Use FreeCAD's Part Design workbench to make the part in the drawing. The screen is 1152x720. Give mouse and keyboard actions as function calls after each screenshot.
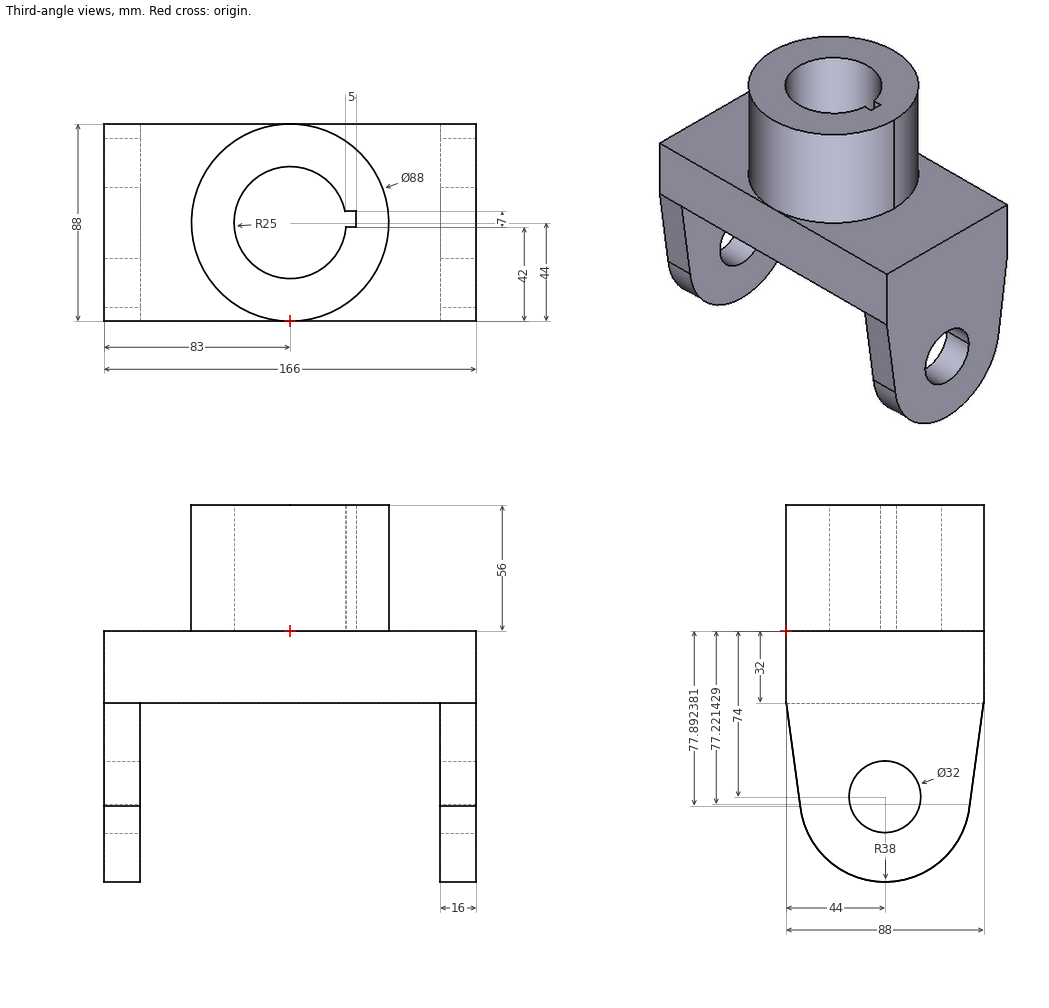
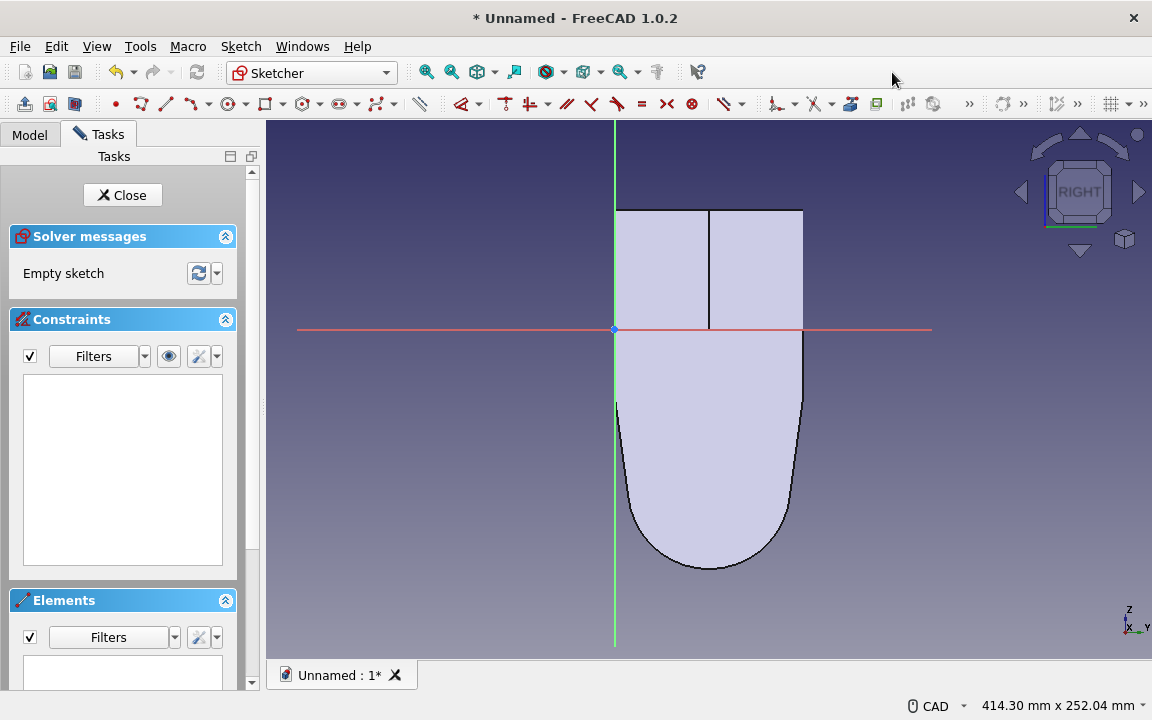
scroll(726, 513, up, 8)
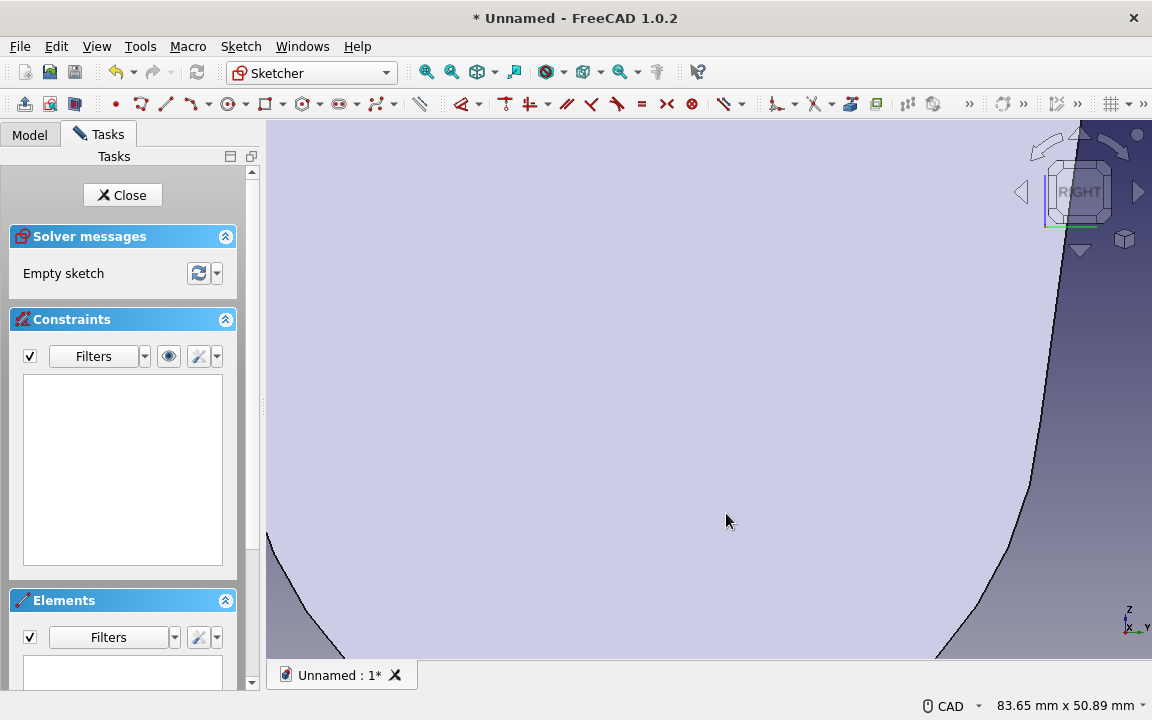
click(228, 104)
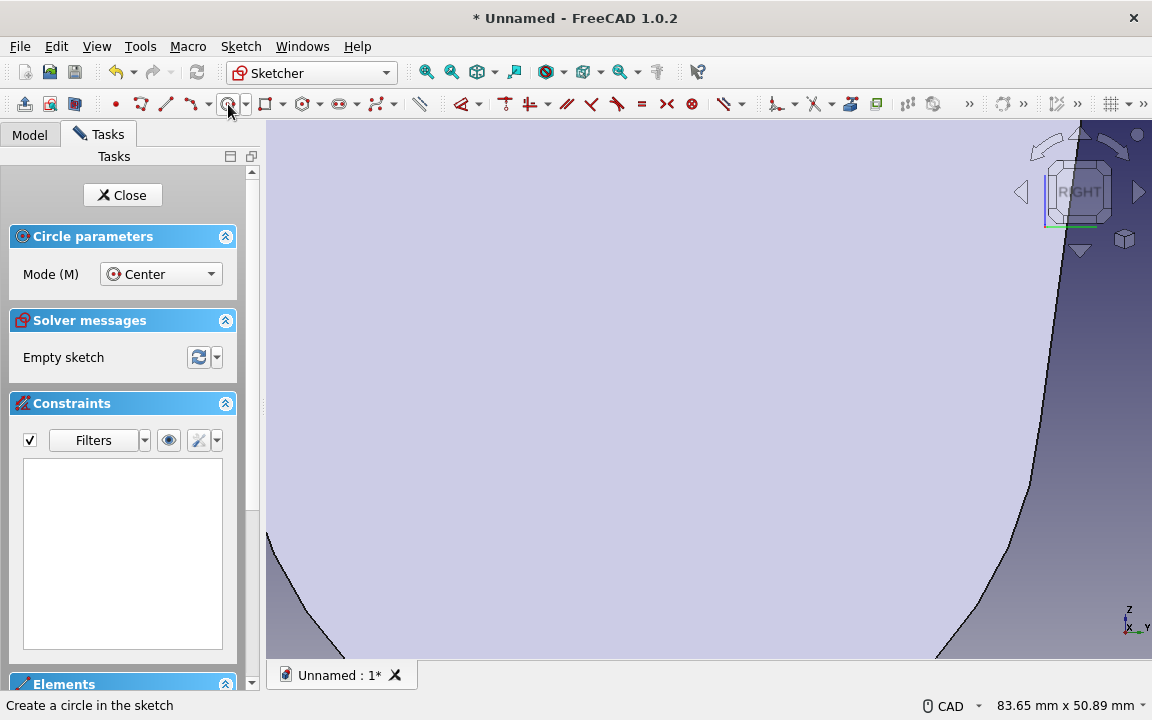
click(640, 386)
move(760, 266)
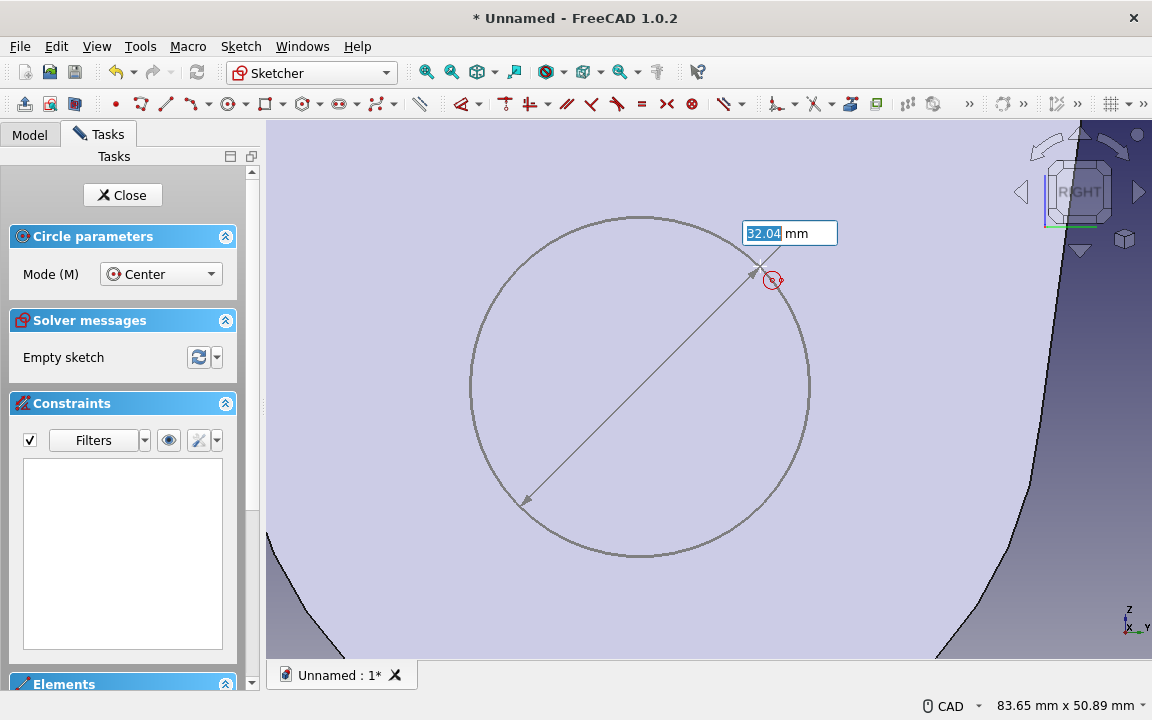
text(32)
key(Return)
key(Escape)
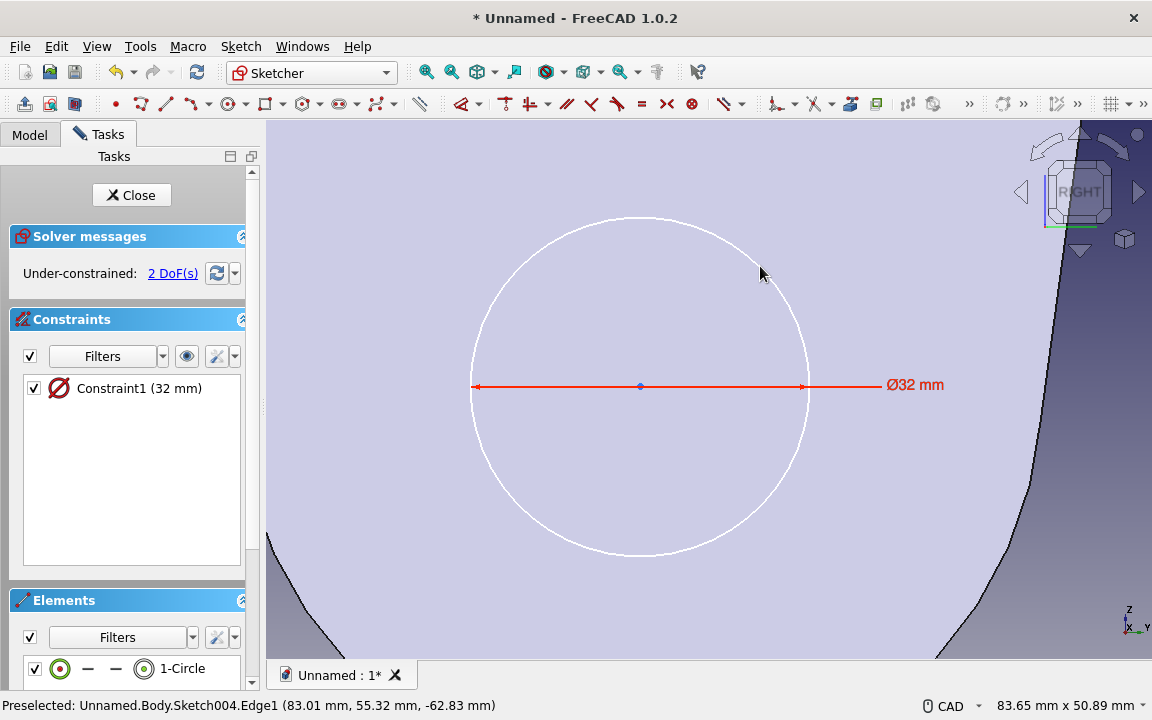
click(460, 104)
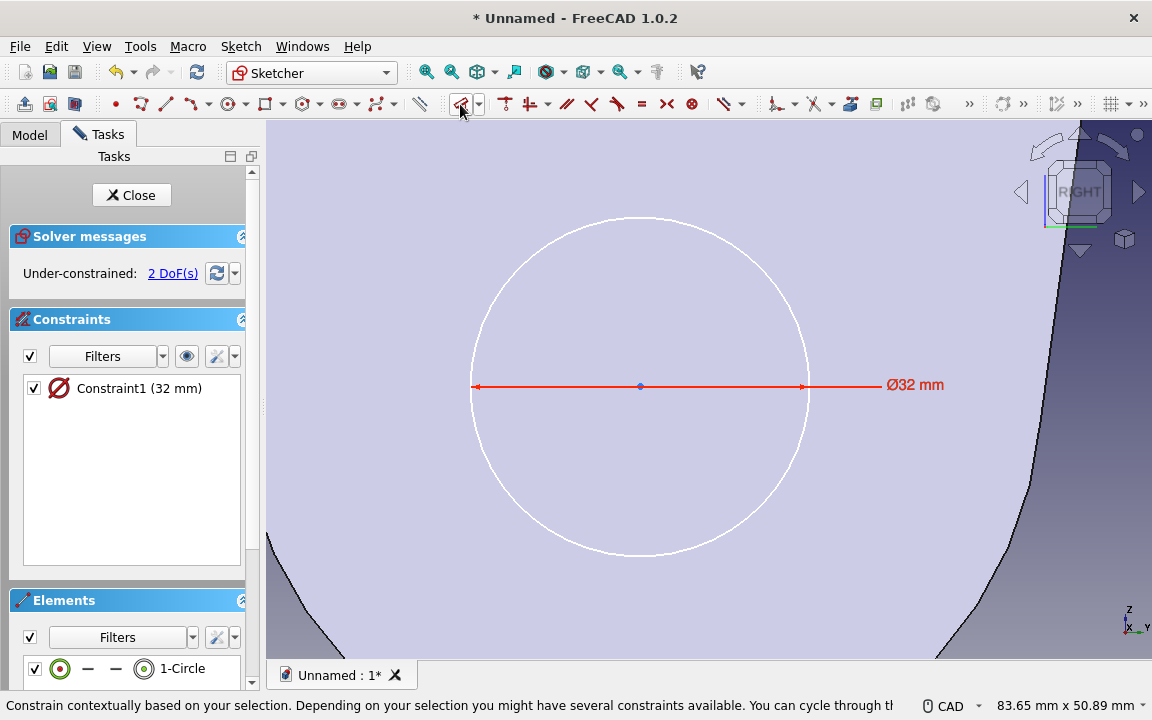
click(640, 387)
click(387, 421)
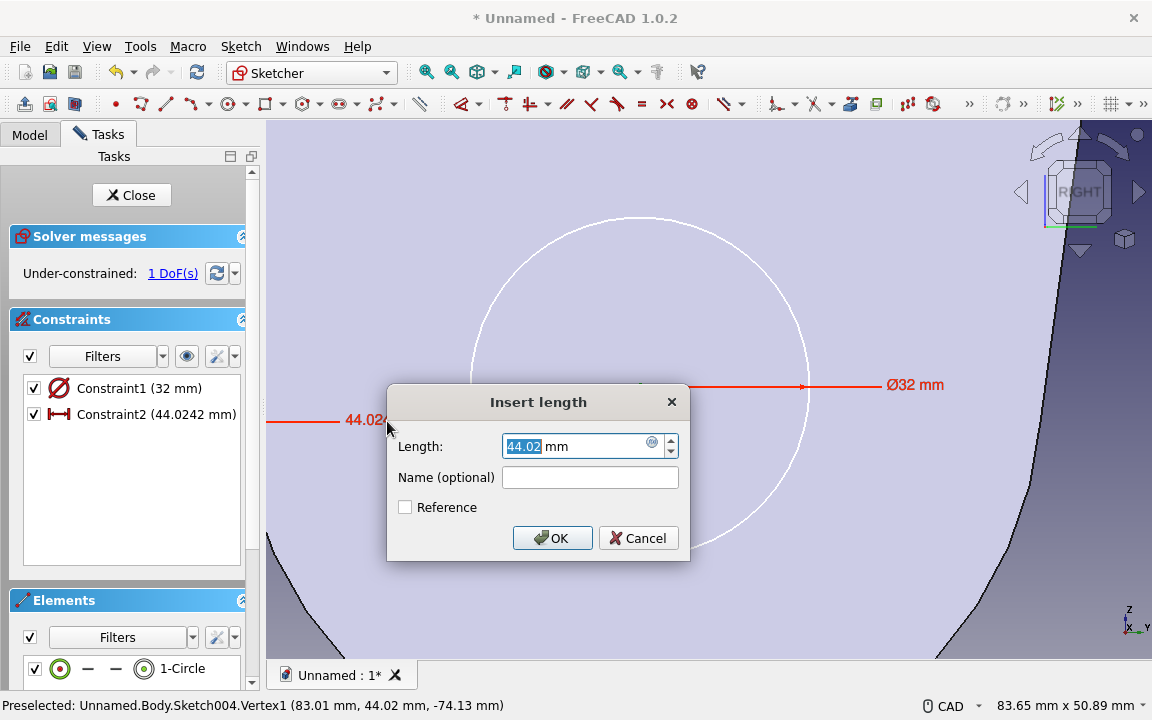
text(44)
key(Return)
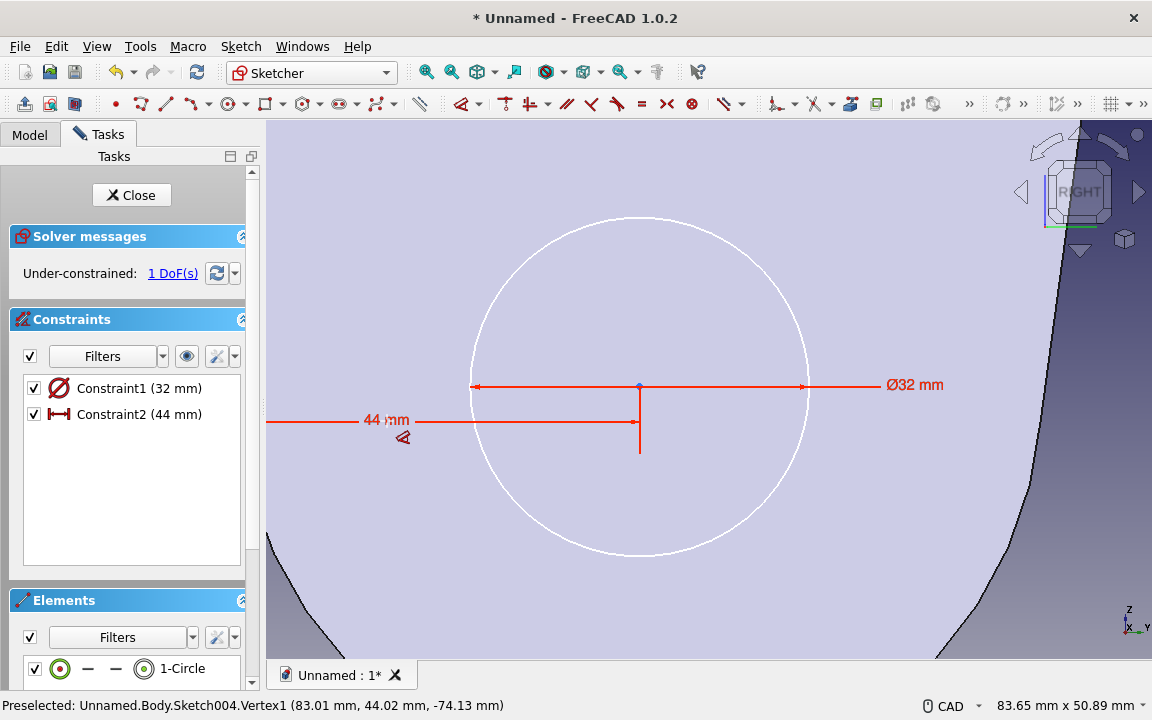
click(640, 387)
click(674, 268)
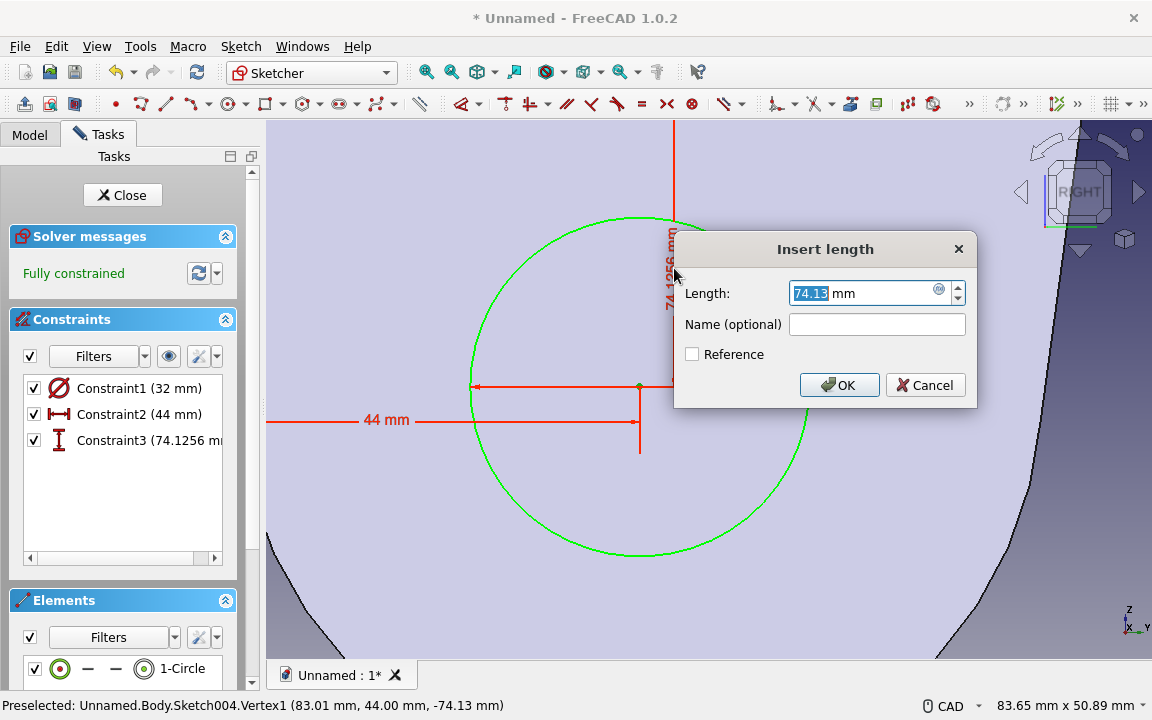
text(74)
key(Return)
key(Escape)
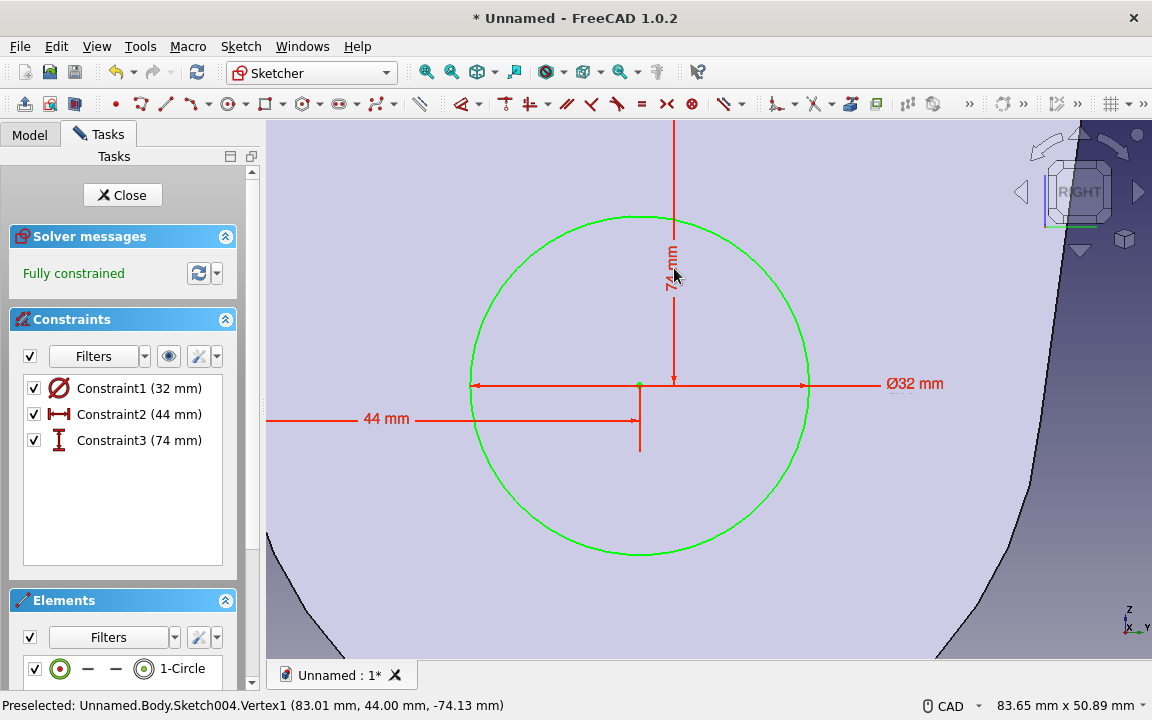
click(123, 195)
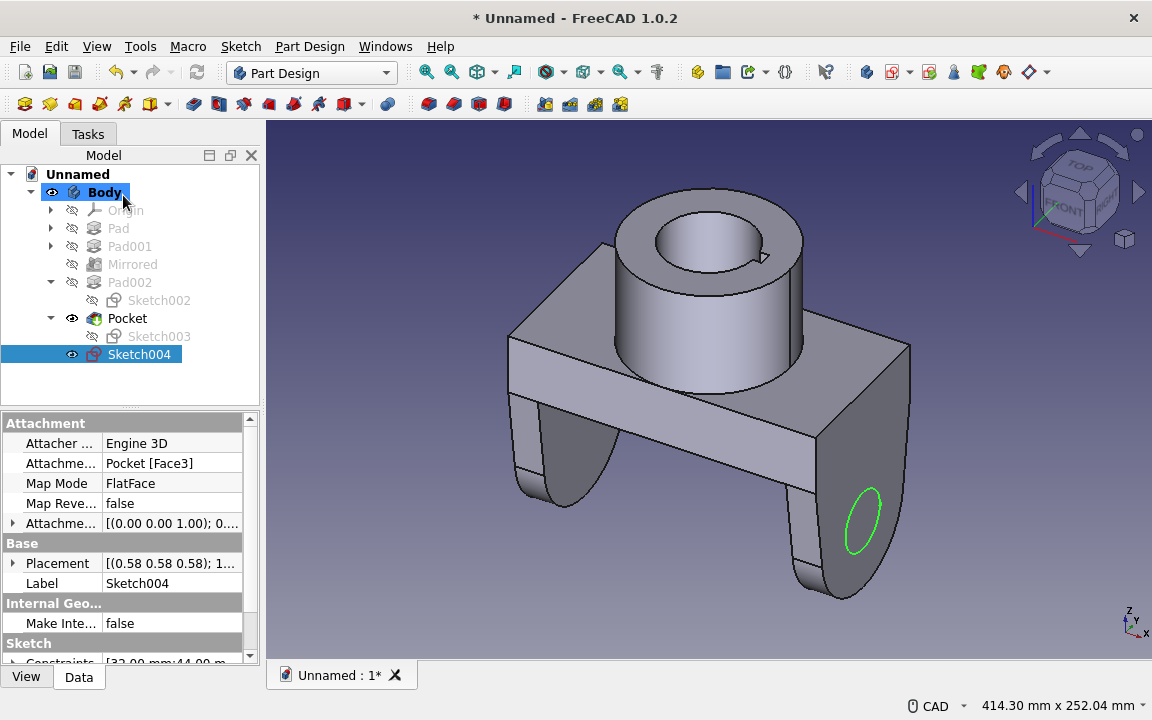
click(194, 104)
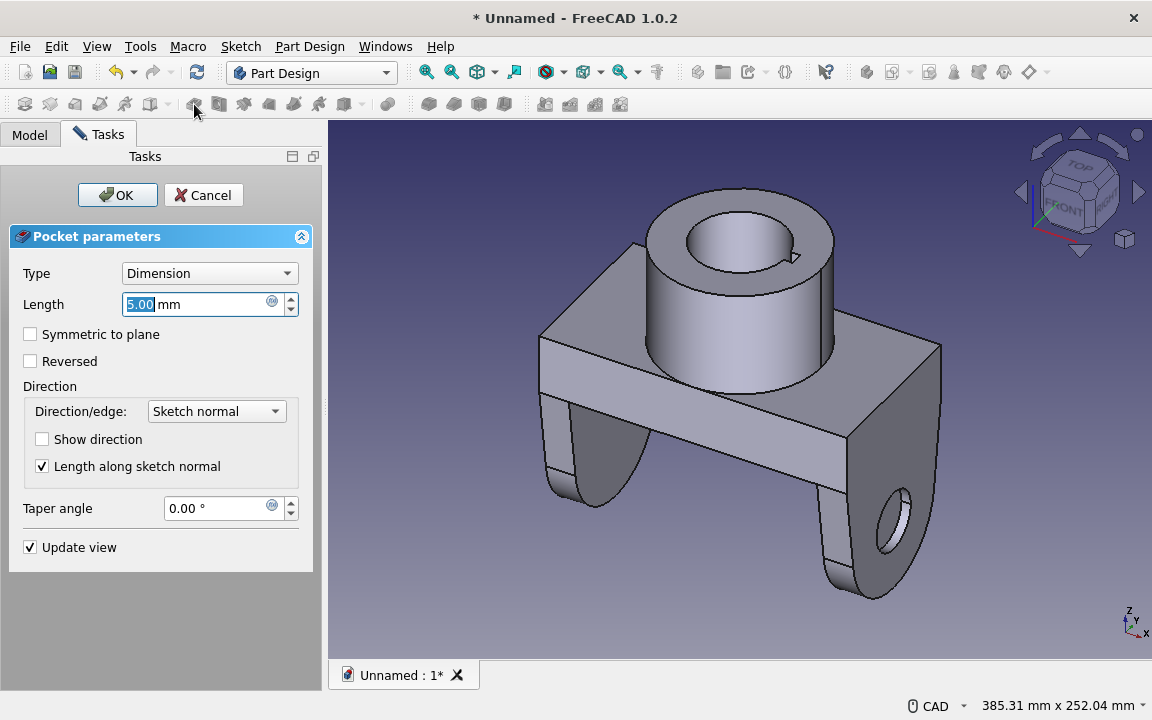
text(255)
key(Tab)